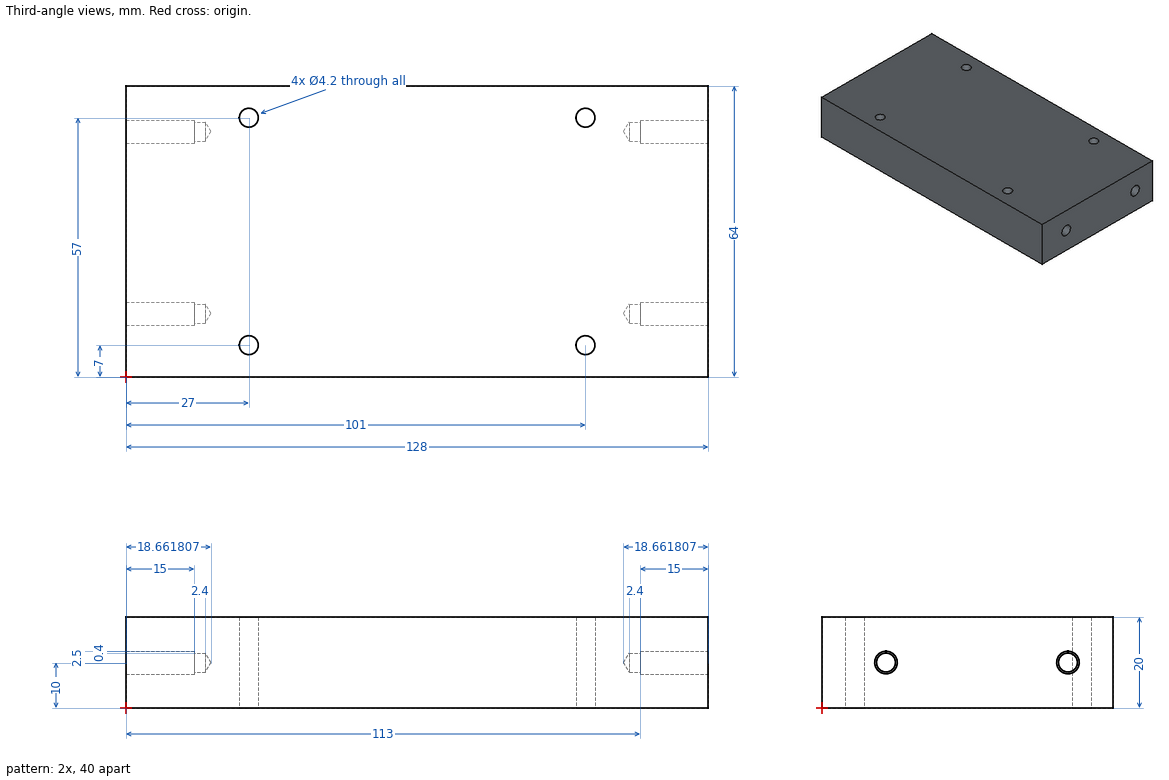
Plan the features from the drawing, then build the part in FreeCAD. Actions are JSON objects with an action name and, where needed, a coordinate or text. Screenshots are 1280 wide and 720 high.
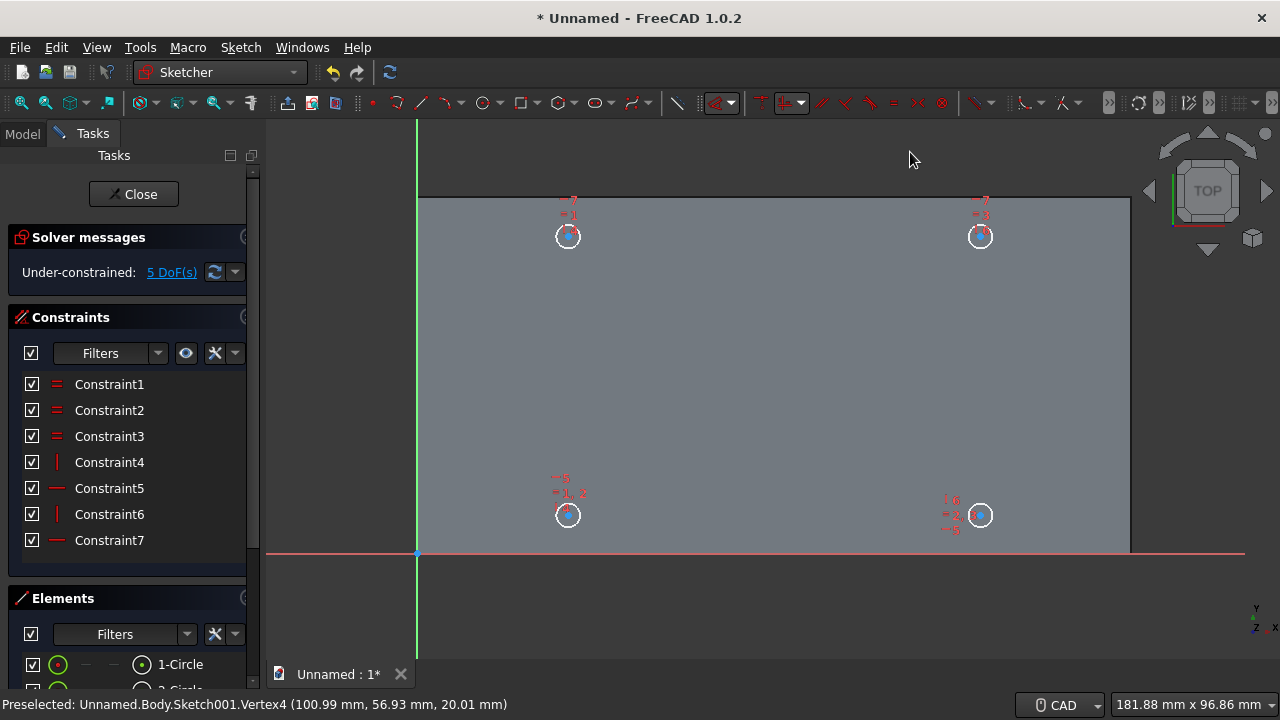
{"action": "scroll", "coordinate": [576, 228], "scroll_direction": "up", "scroll_amount": 3}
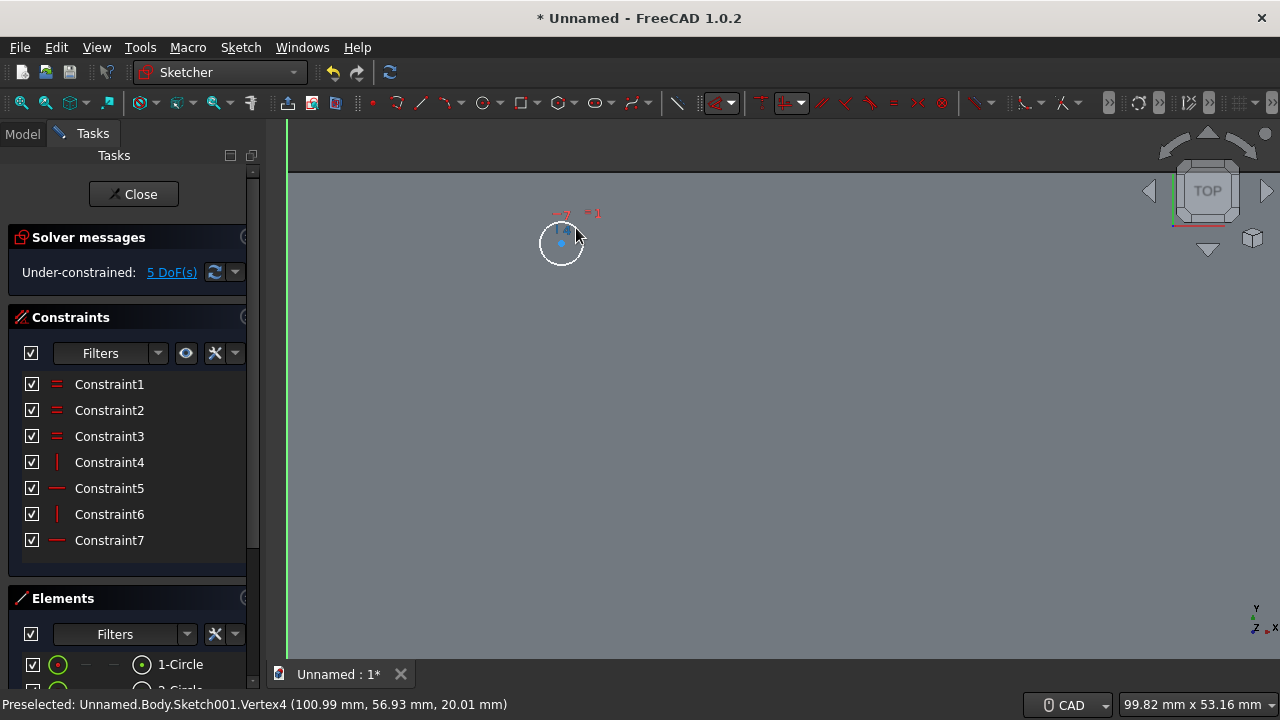
{"action": "left_click", "coordinate": [577, 228]}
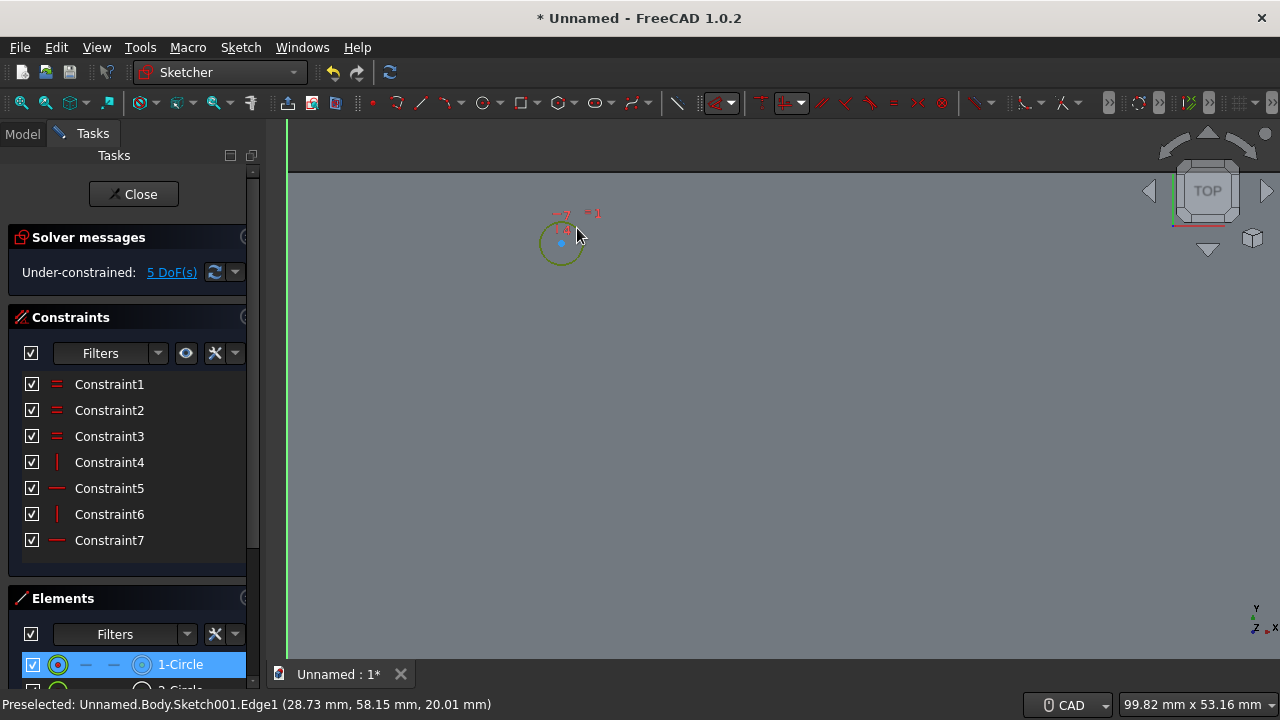
{"action": "key", "text": "k o"}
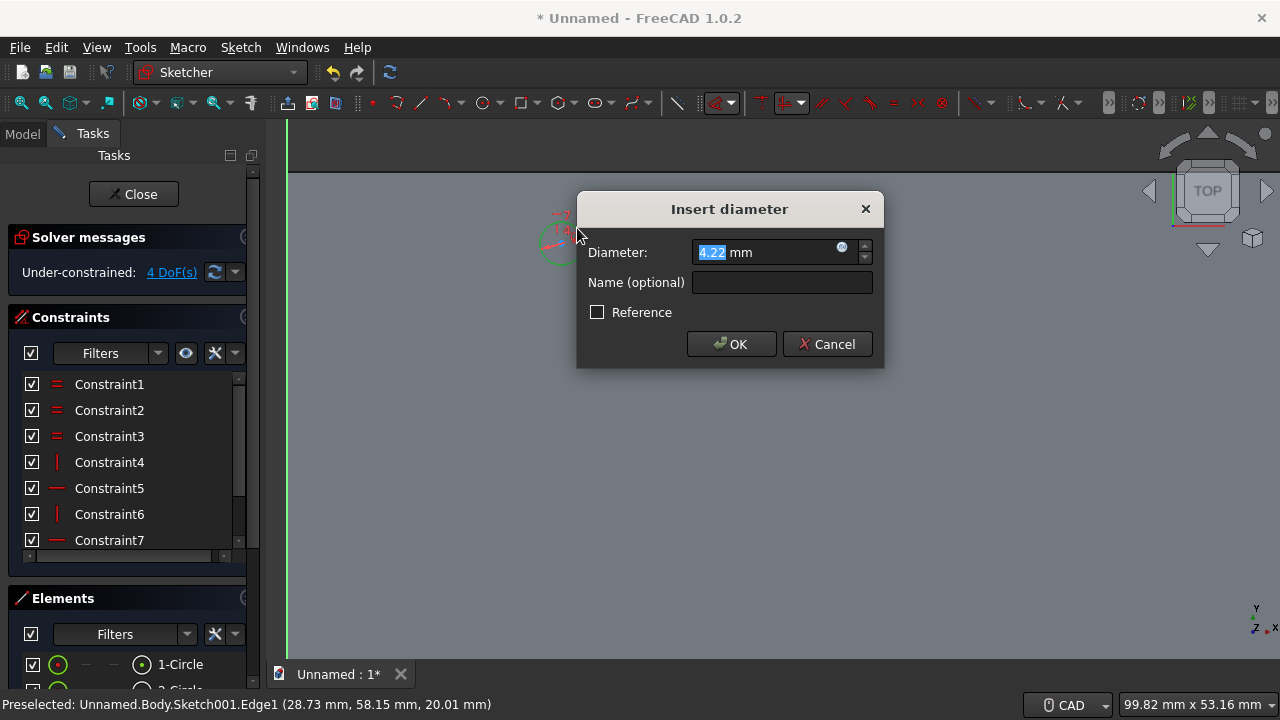
{"action": "type", "text": "4.2"}
{"action": "key", "text": "Return"}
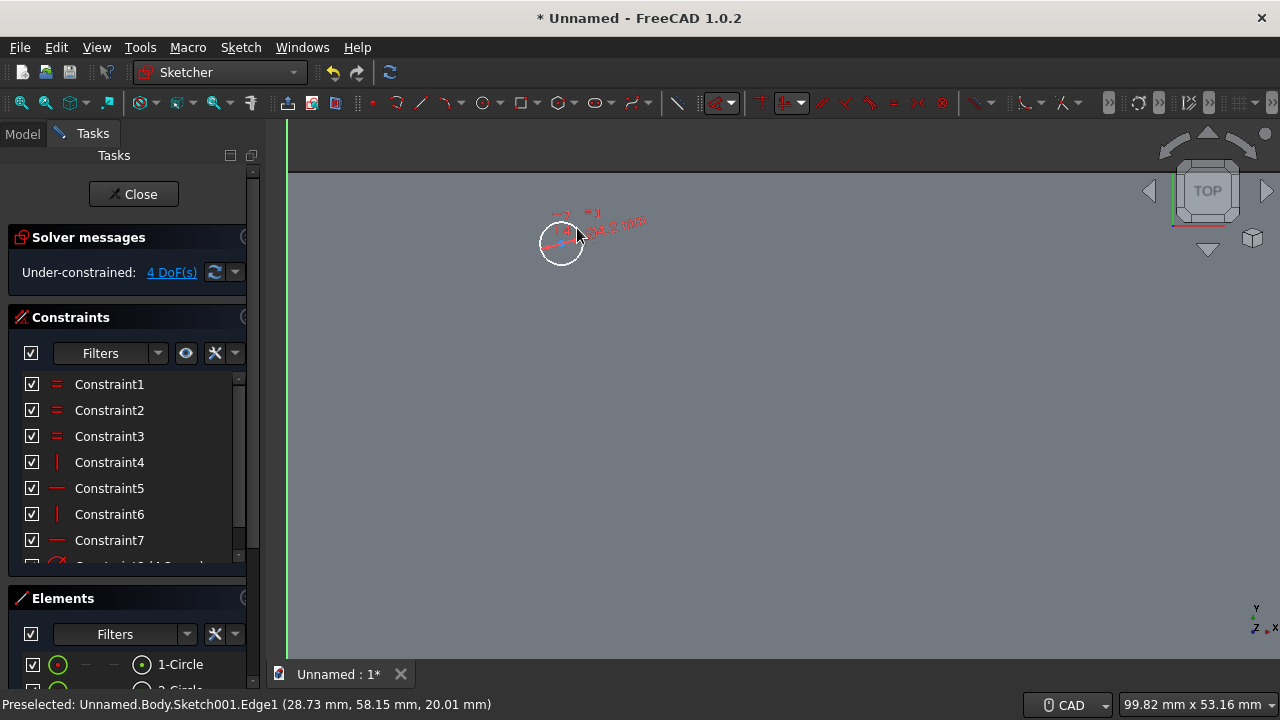
{"action": "scroll", "coordinate": [575, 228], "scroll_direction": "down", "scroll_amount": 3}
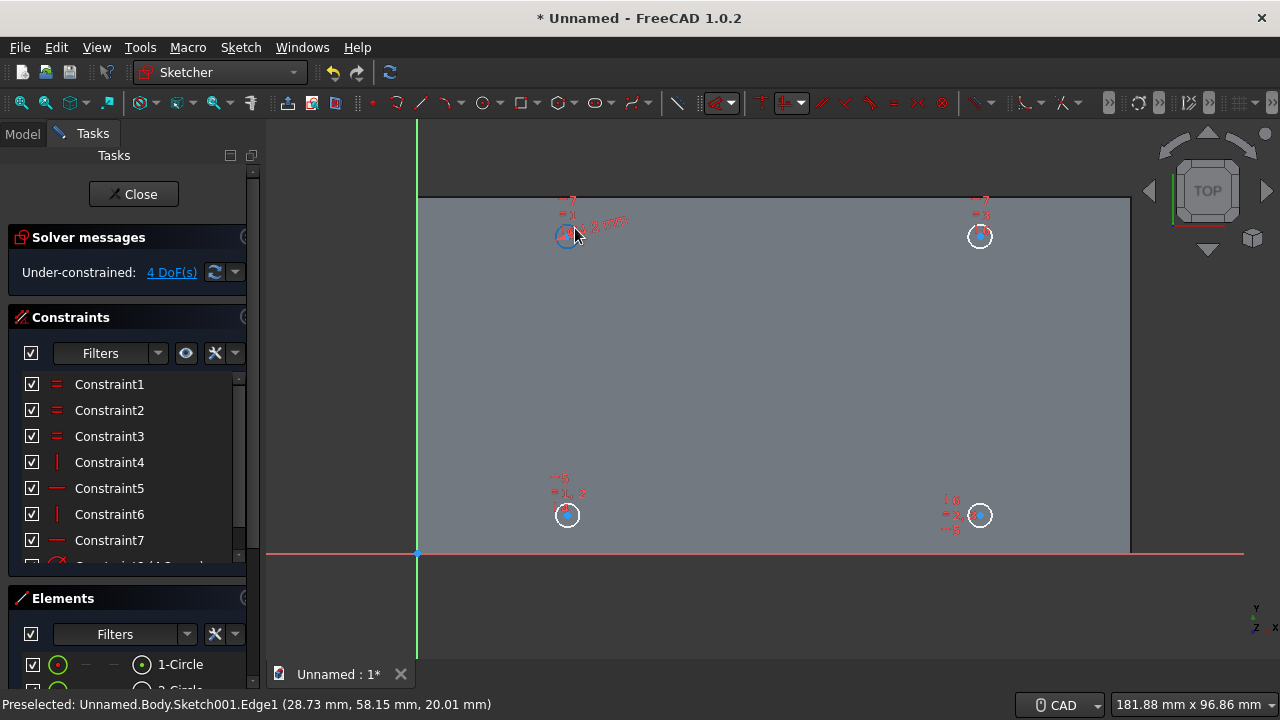
{"action": "left_click", "coordinate": [568, 515]}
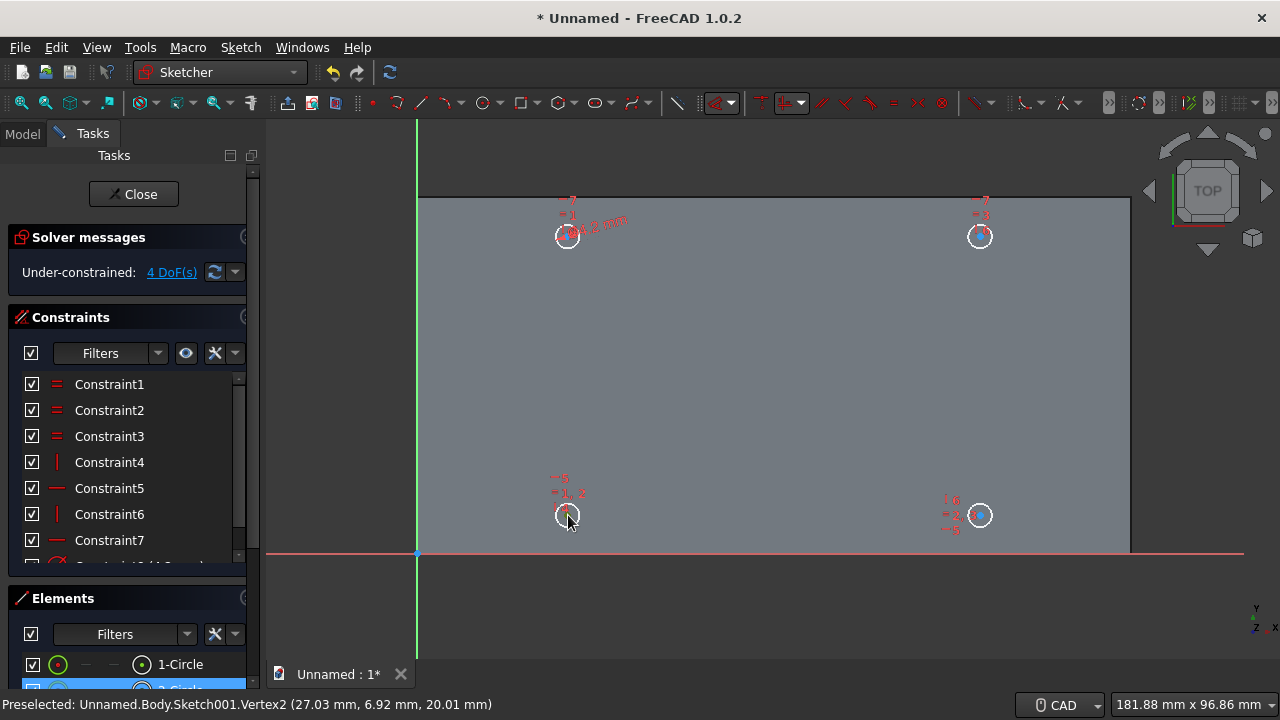
{"action": "left_click", "coordinate": [734, 104]}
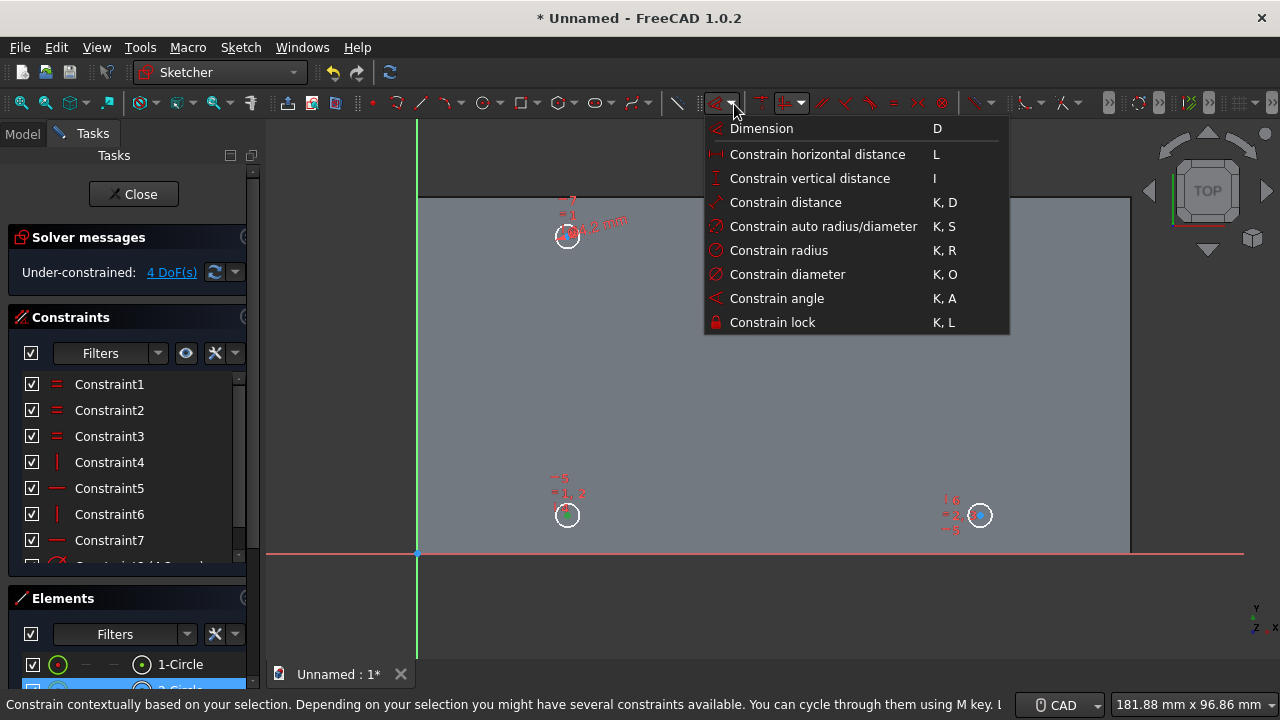
{"action": "left_click", "coordinate": [857, 178]}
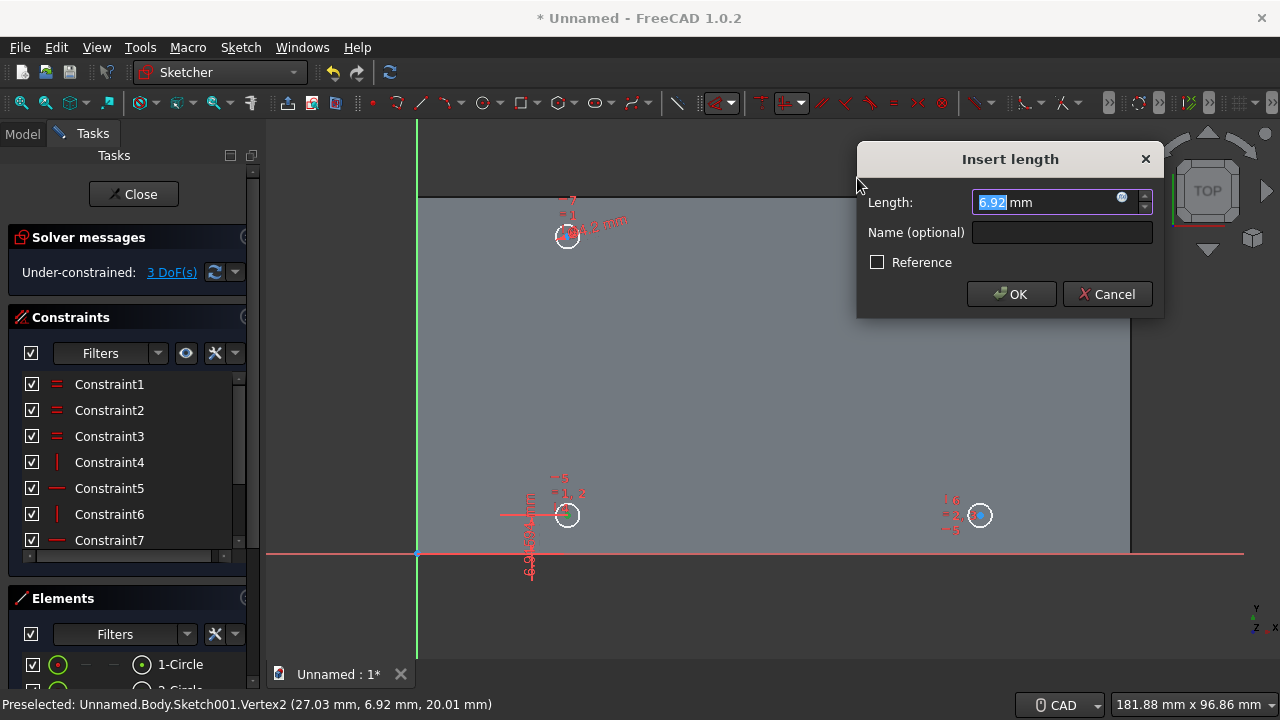
{"action": "type", "text": "7"}
{"action": "key", "text": "Return"}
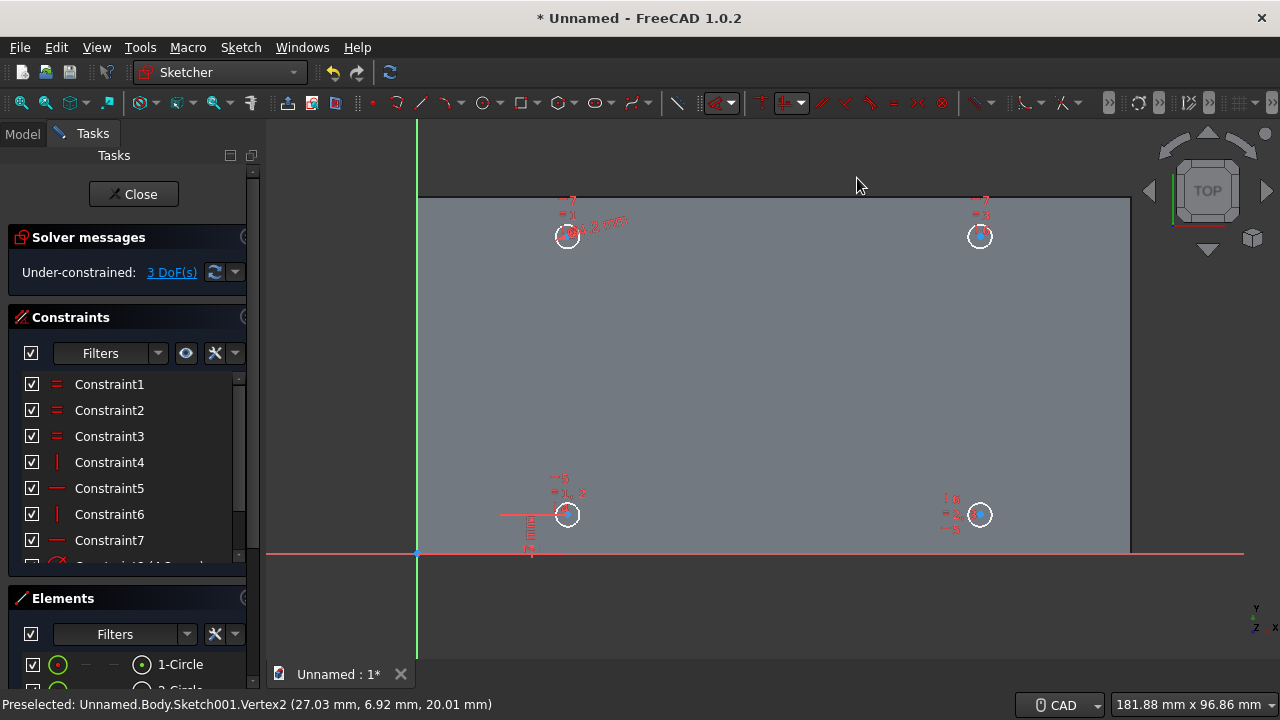
{"action": "left_click", "coordinate": [568, 237]}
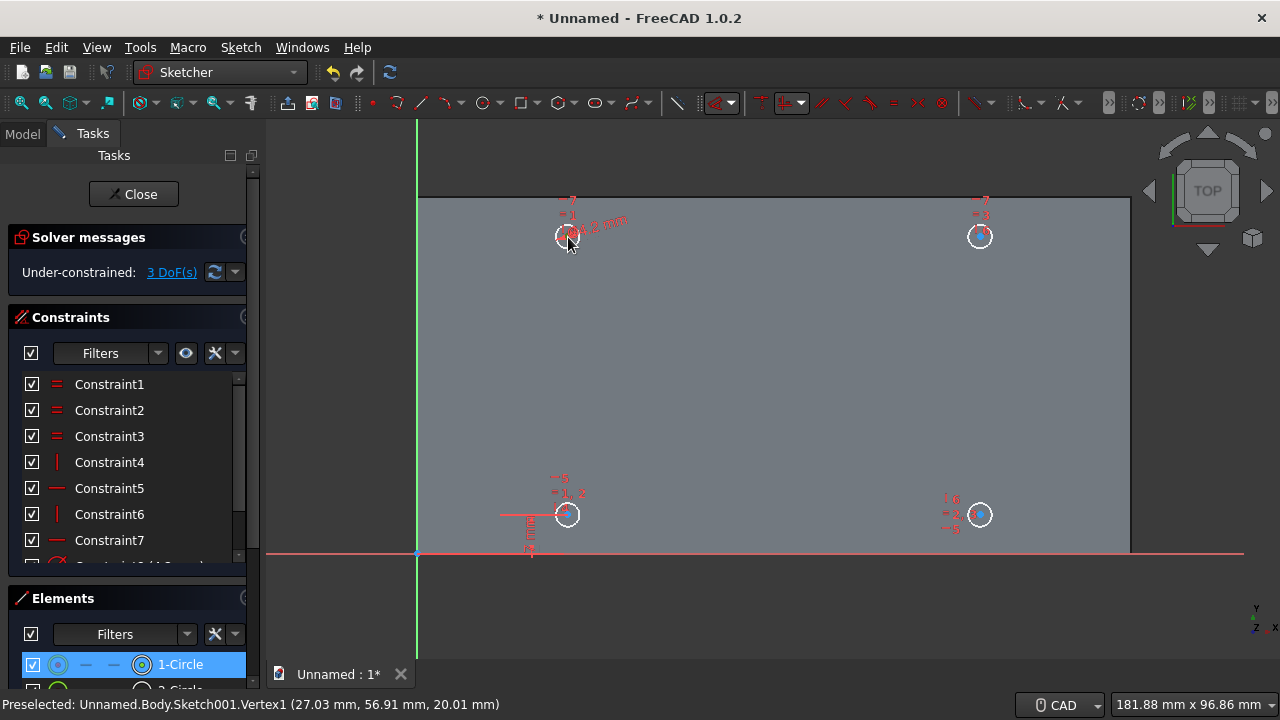
{"action": "left_click", "coordinate": [734, 104]}